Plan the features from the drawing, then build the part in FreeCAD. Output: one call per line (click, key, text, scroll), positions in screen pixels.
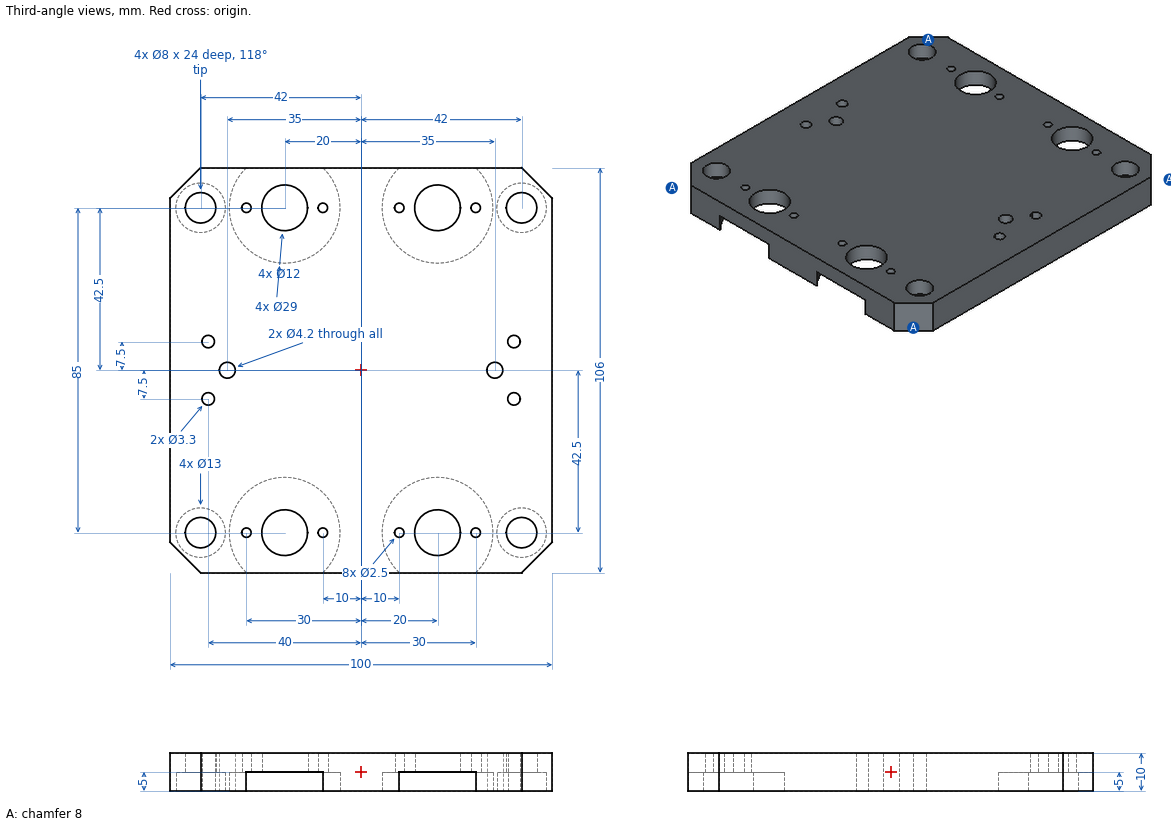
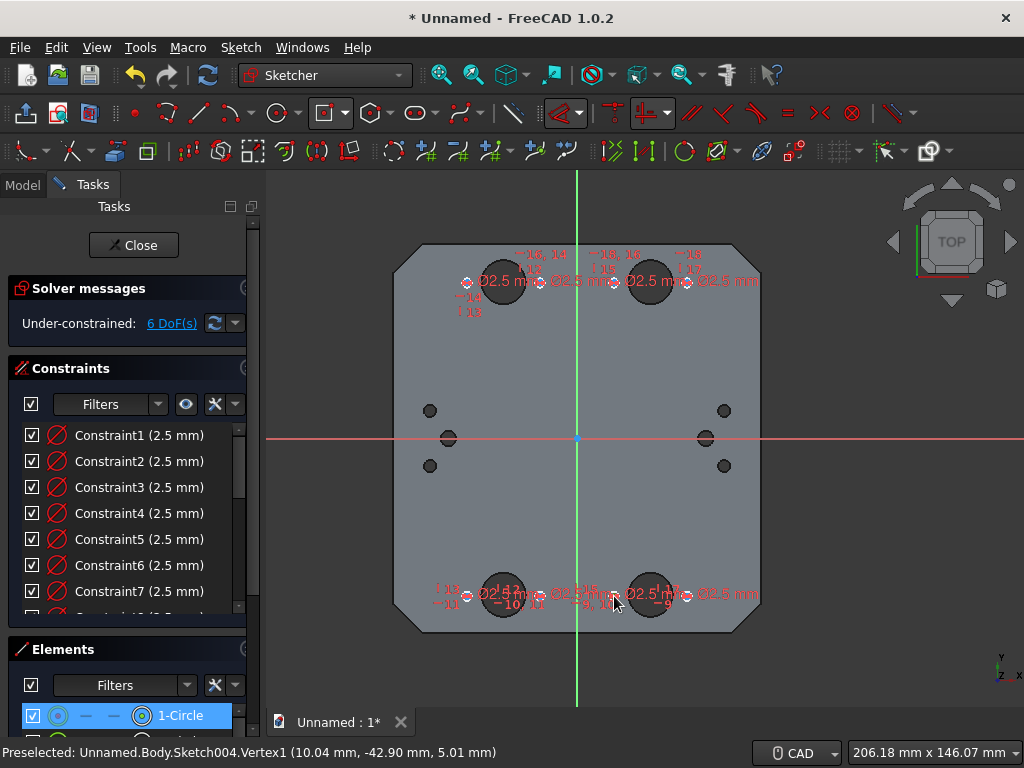
key(l)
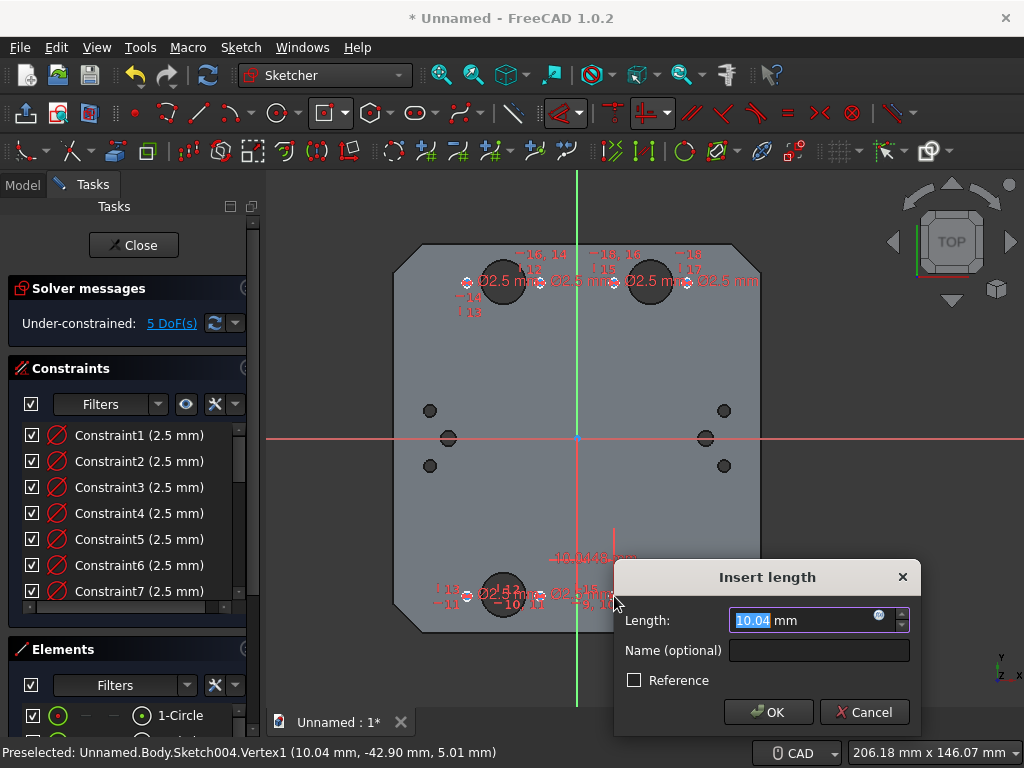
text(10)
key(Return)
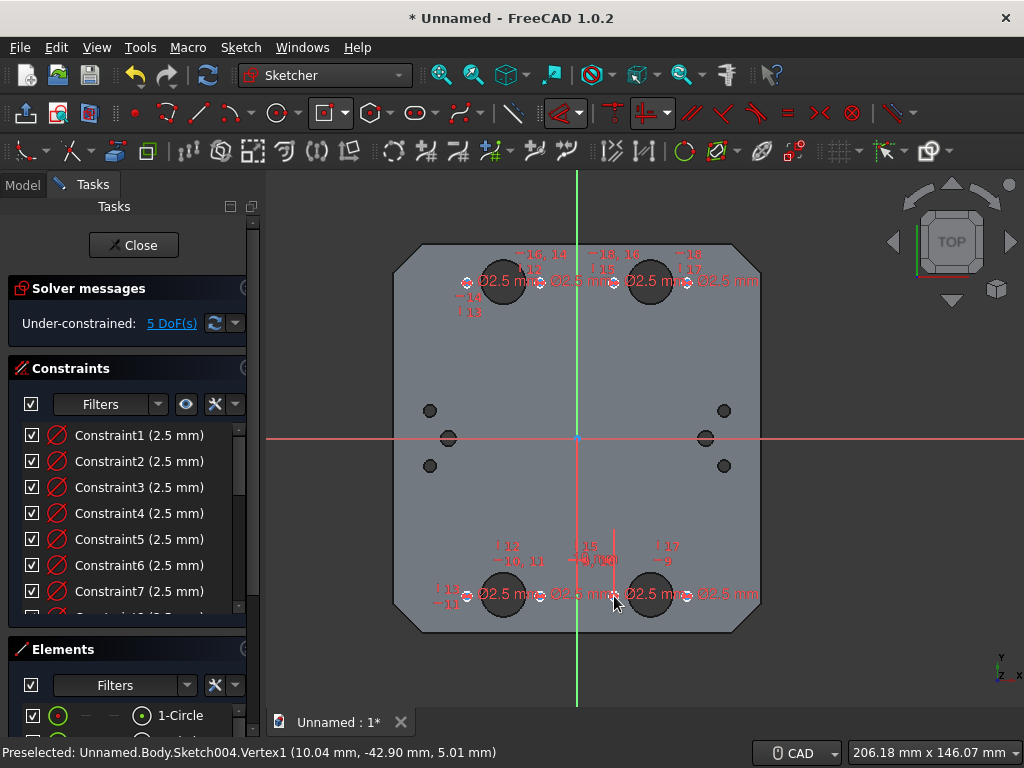
click(687, 596)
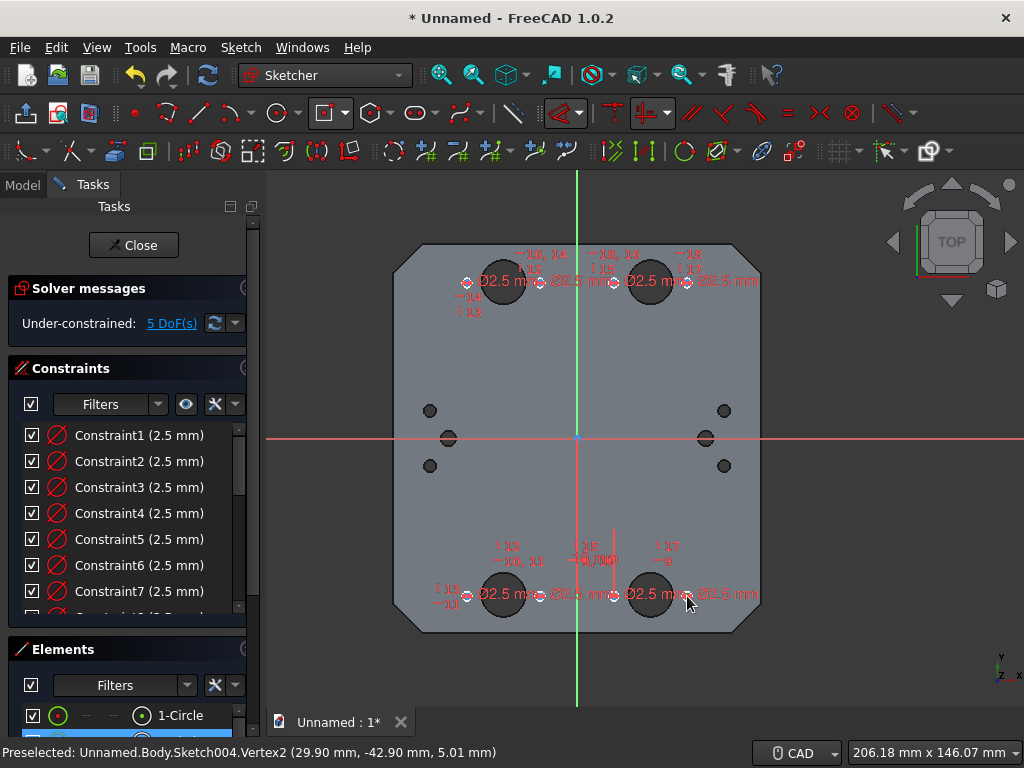
key(l)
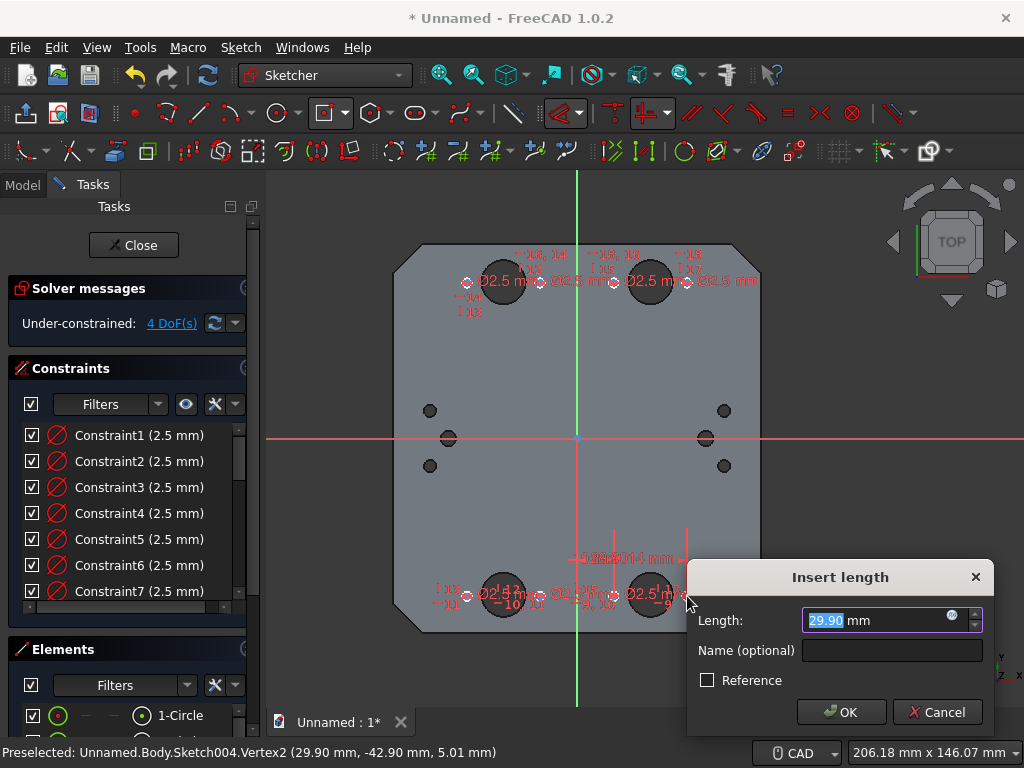
text(30)
key(Return)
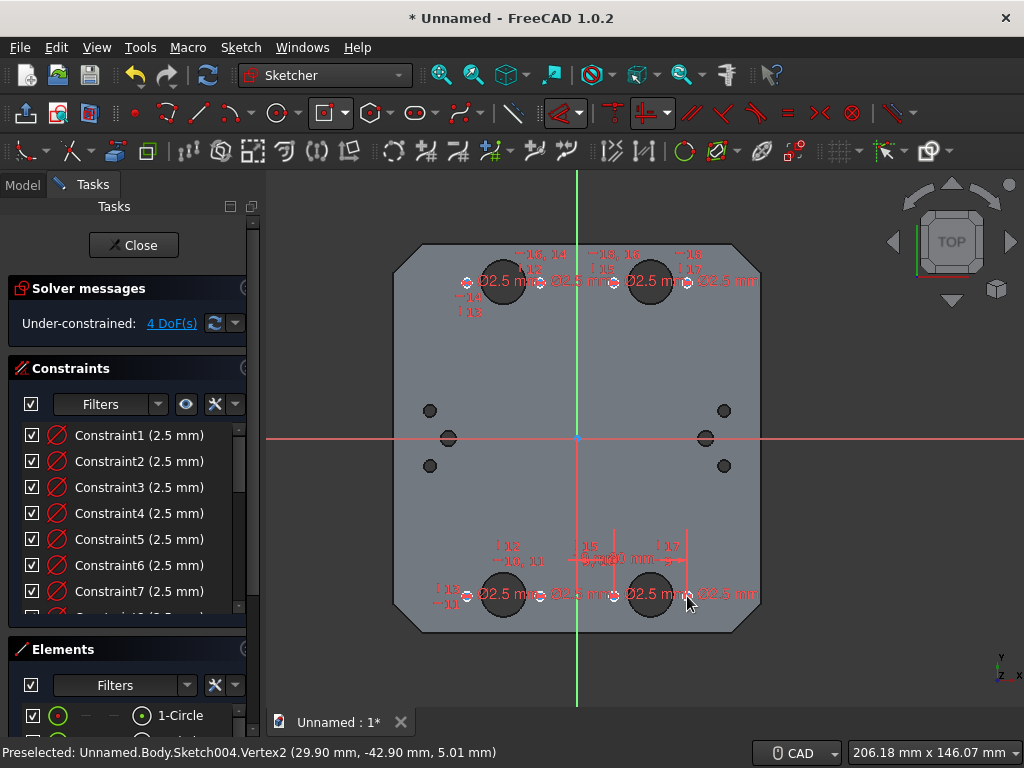
click(540, 596)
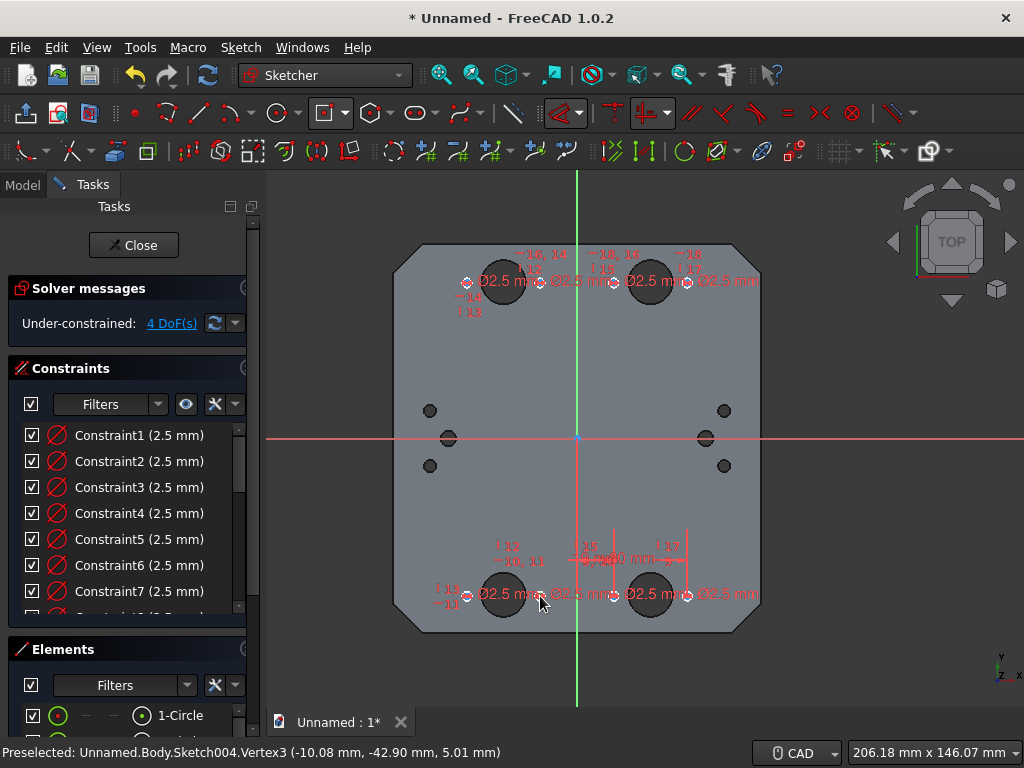
click(582, 114)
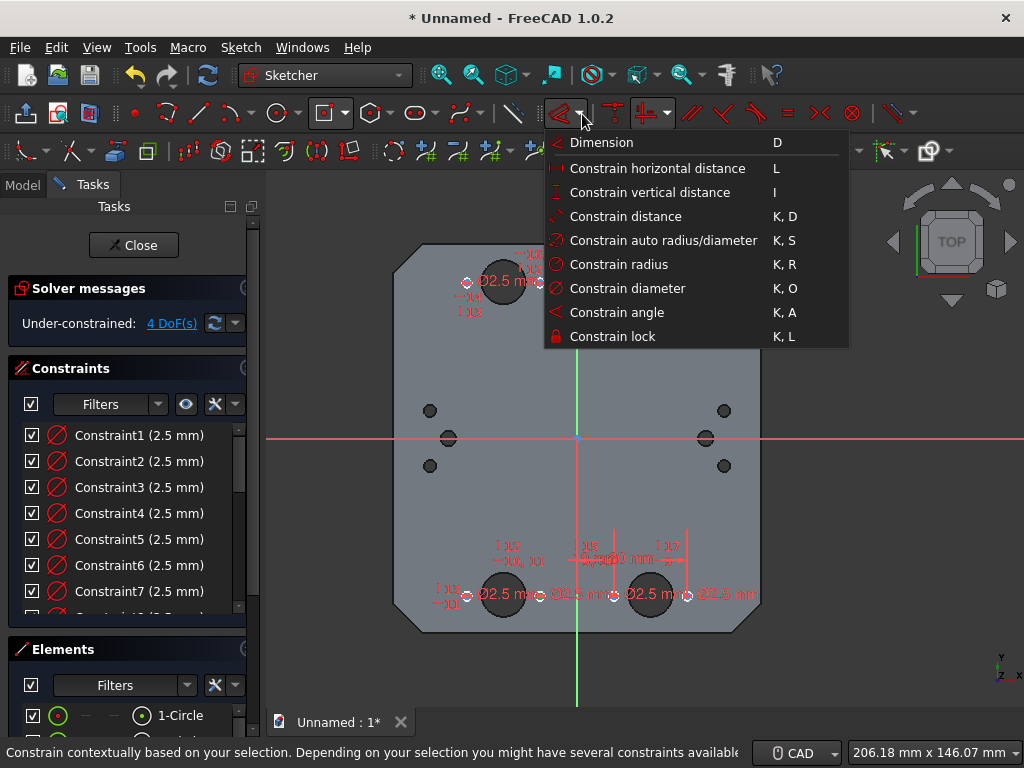
click(697, 168)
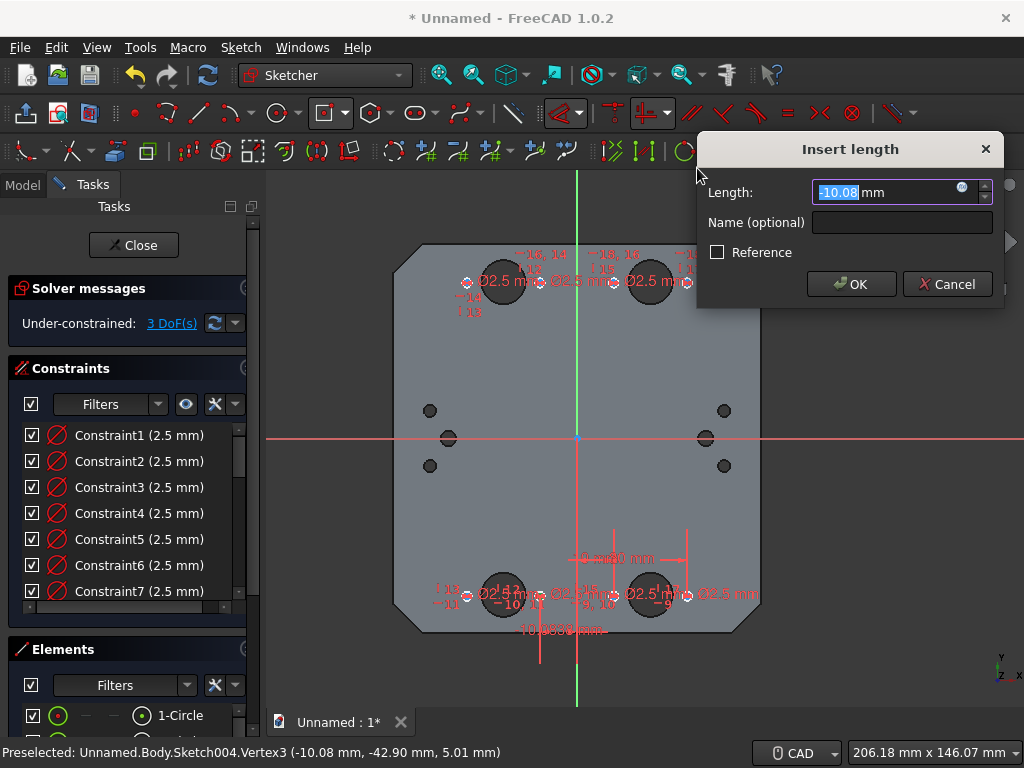
text(-10)
key(Return)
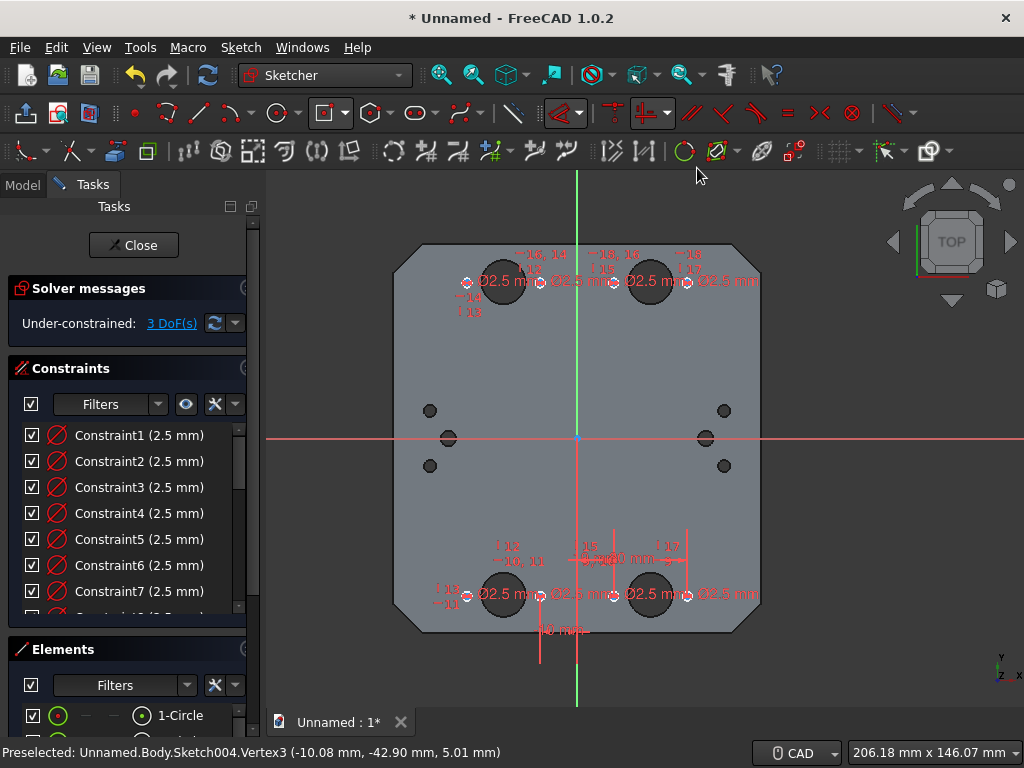
click(467, 596)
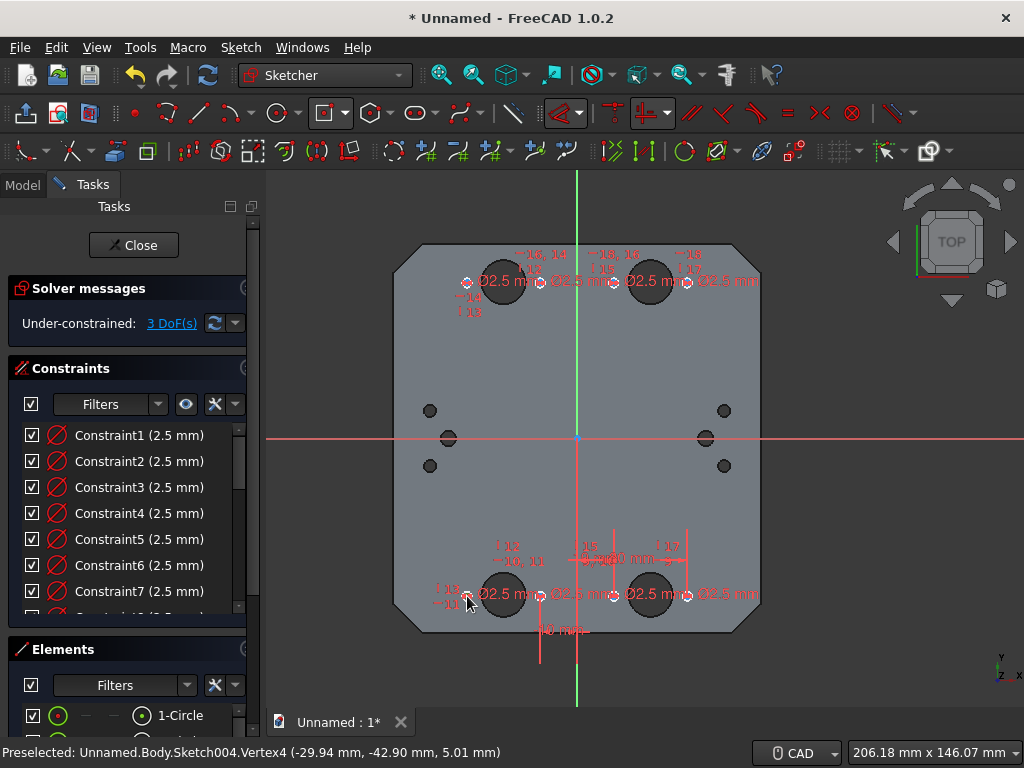
click(582, 114)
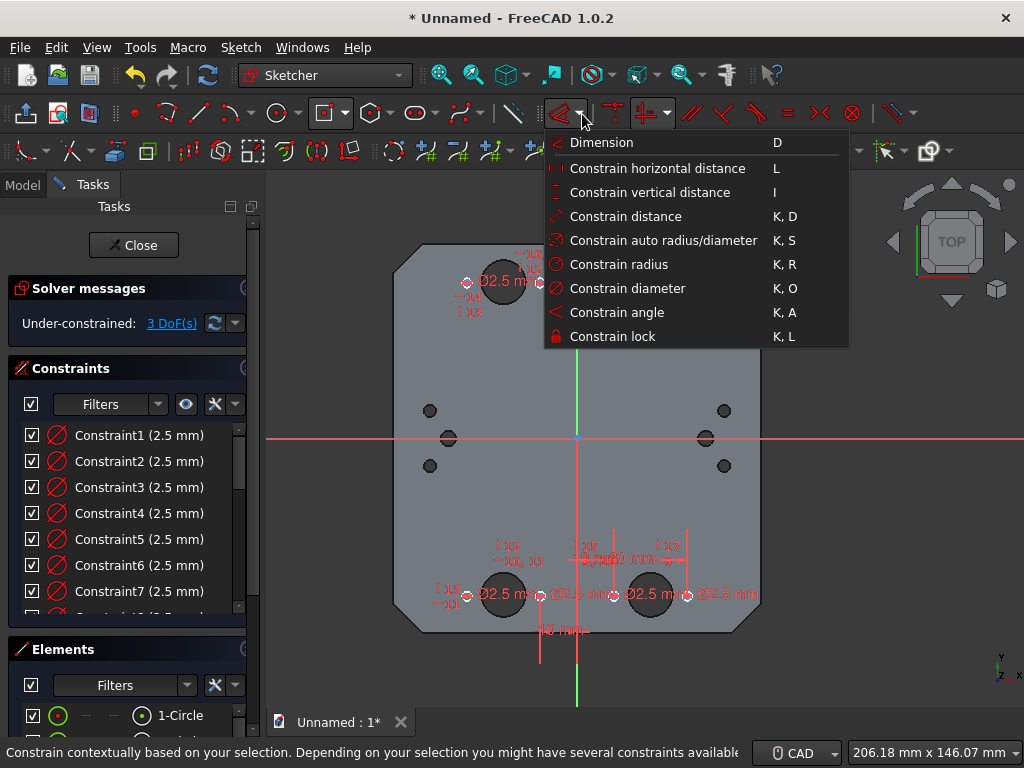
click(697, 168)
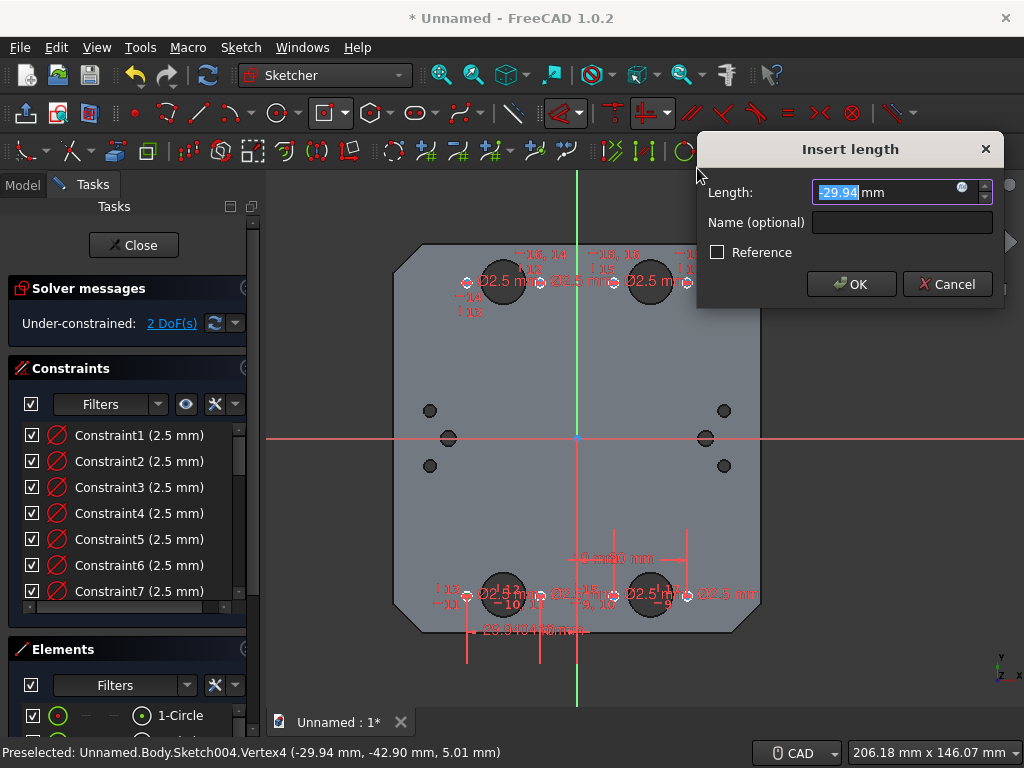
text(-30)
key(Return)